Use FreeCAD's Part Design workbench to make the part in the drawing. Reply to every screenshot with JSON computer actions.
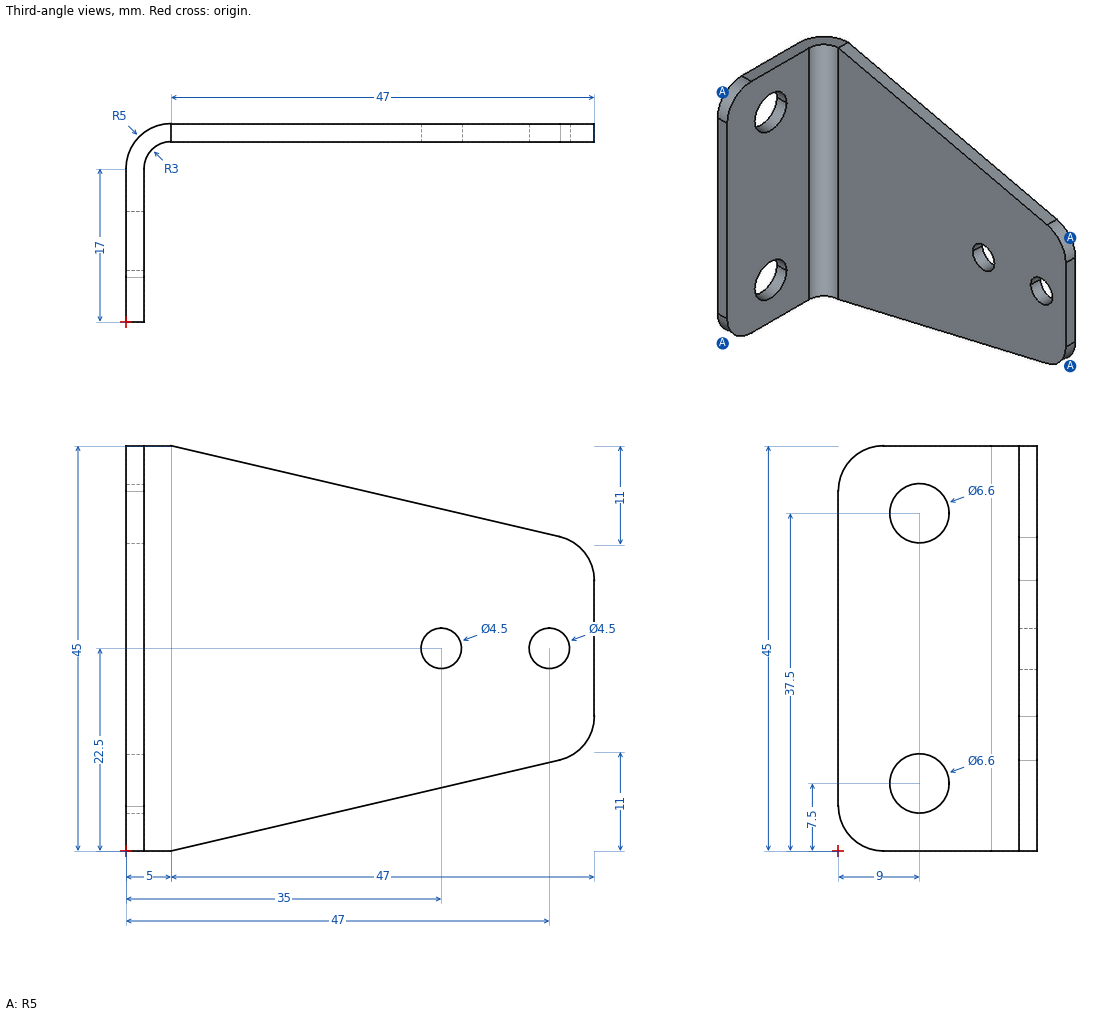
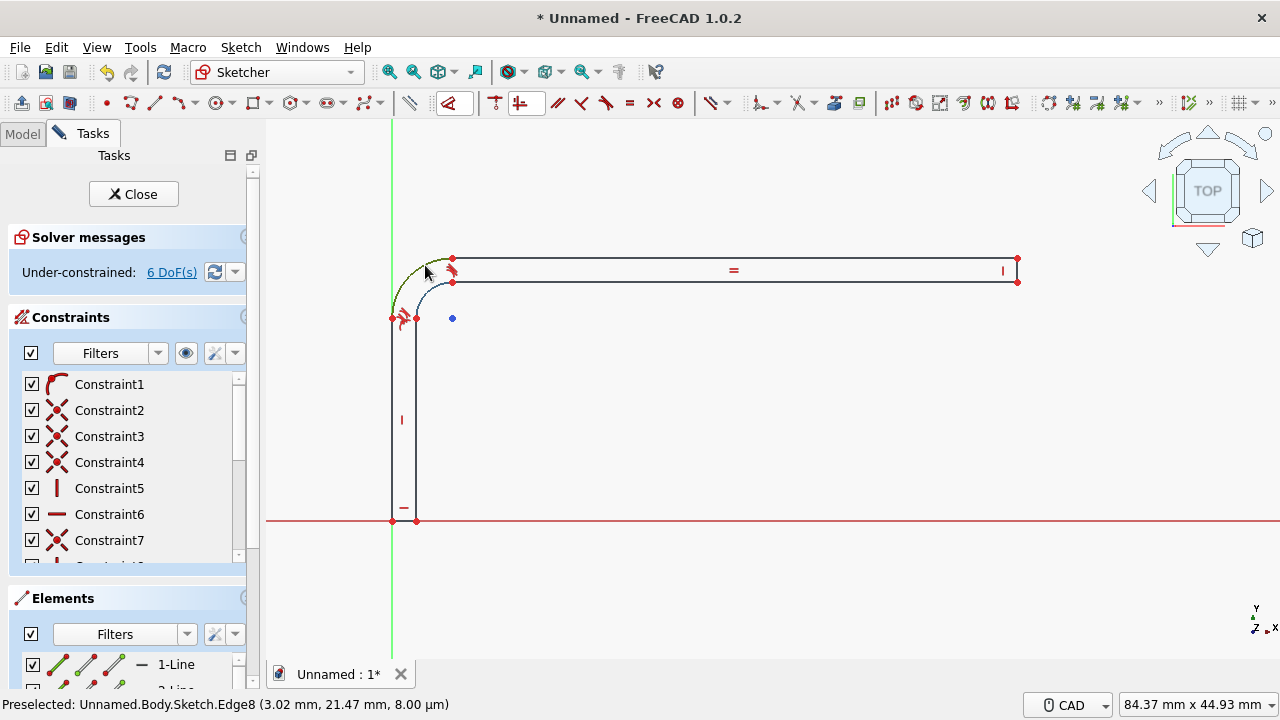
{"action": "key", "text": "c"}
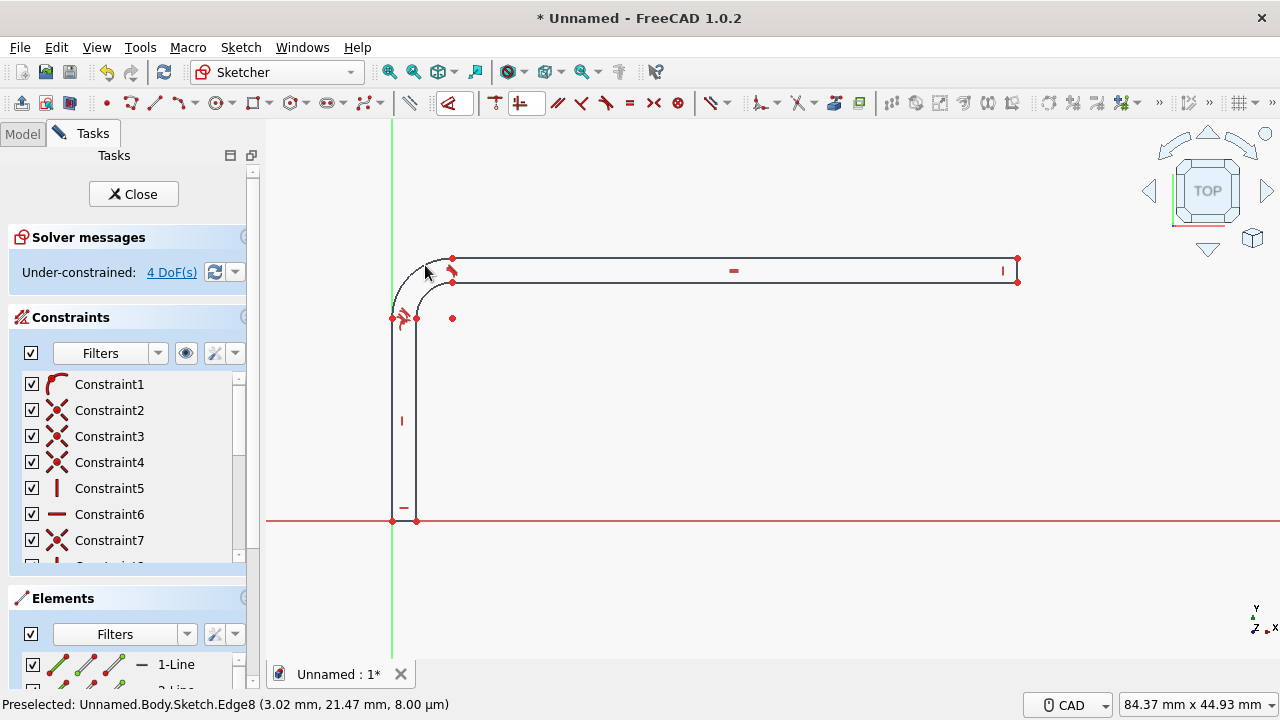
{"action": "left_click", "coordinate": [448, 104]}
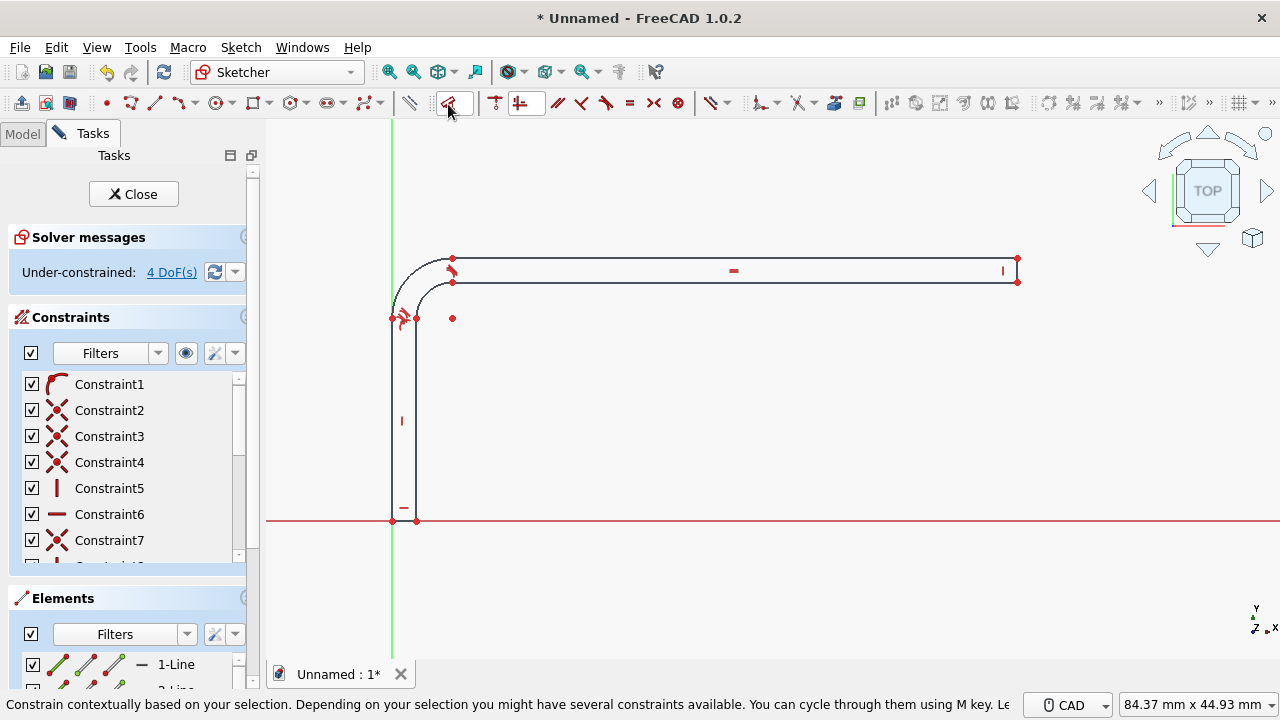
{"action": "left_click", "coordinate": [436, 287]}
{"action": "left_click", "coordinate": [484, 379]}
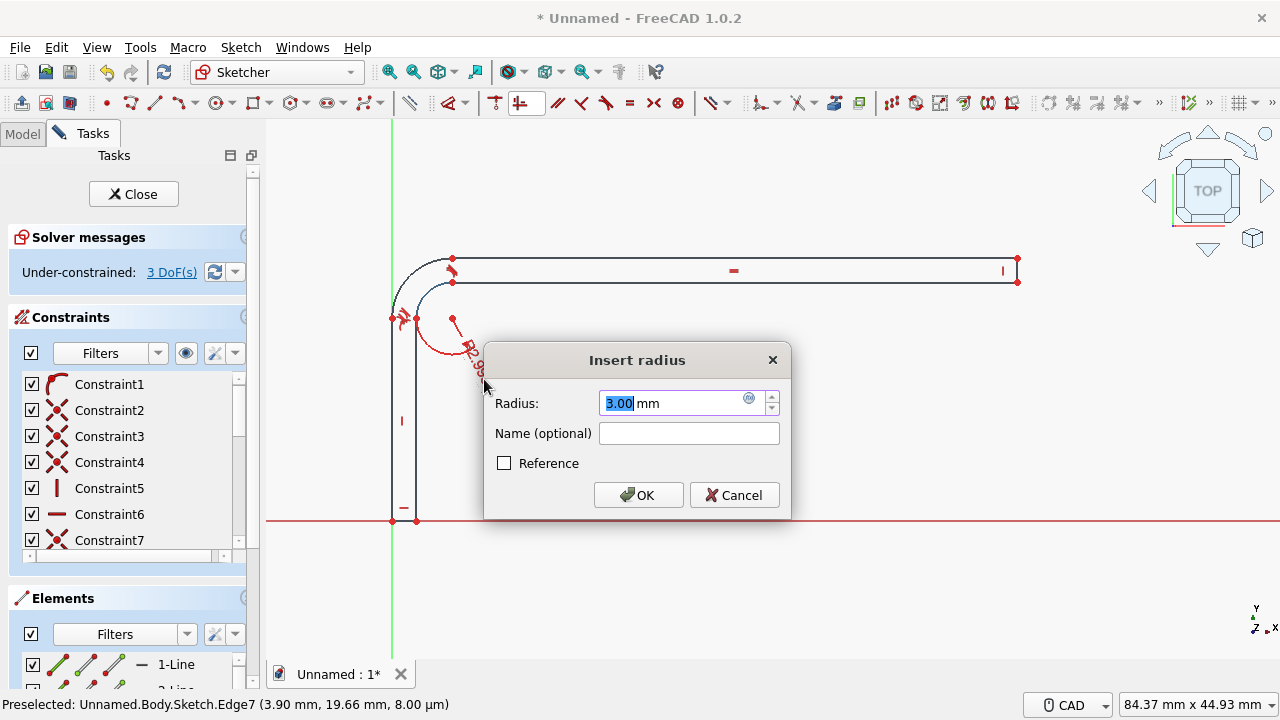
{"action": "type", "text": "3"}
{"action": "key", "text": "Return"}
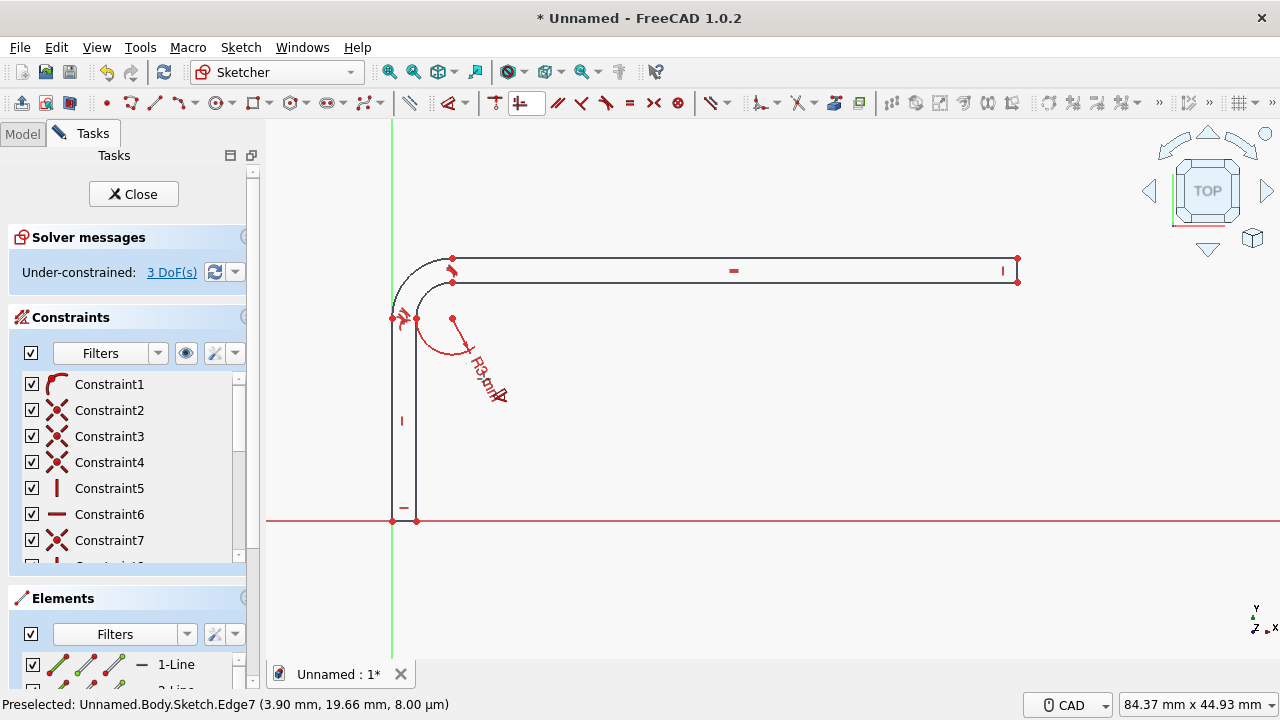
{"action": "left_click", "coordinate": [425, 265]}
{"action": "left_click", "coordinate": [410, 236]}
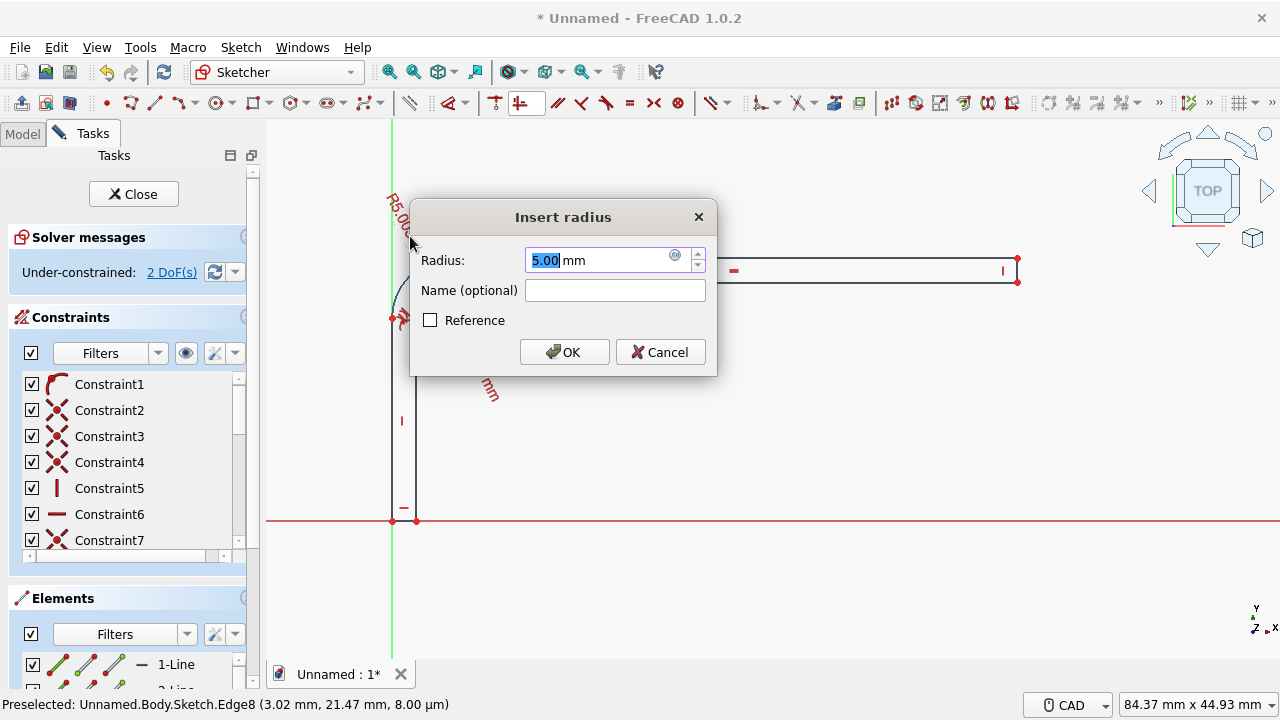
{"action": "type", "text": "5"}
{"action": "key", "text": "Return"}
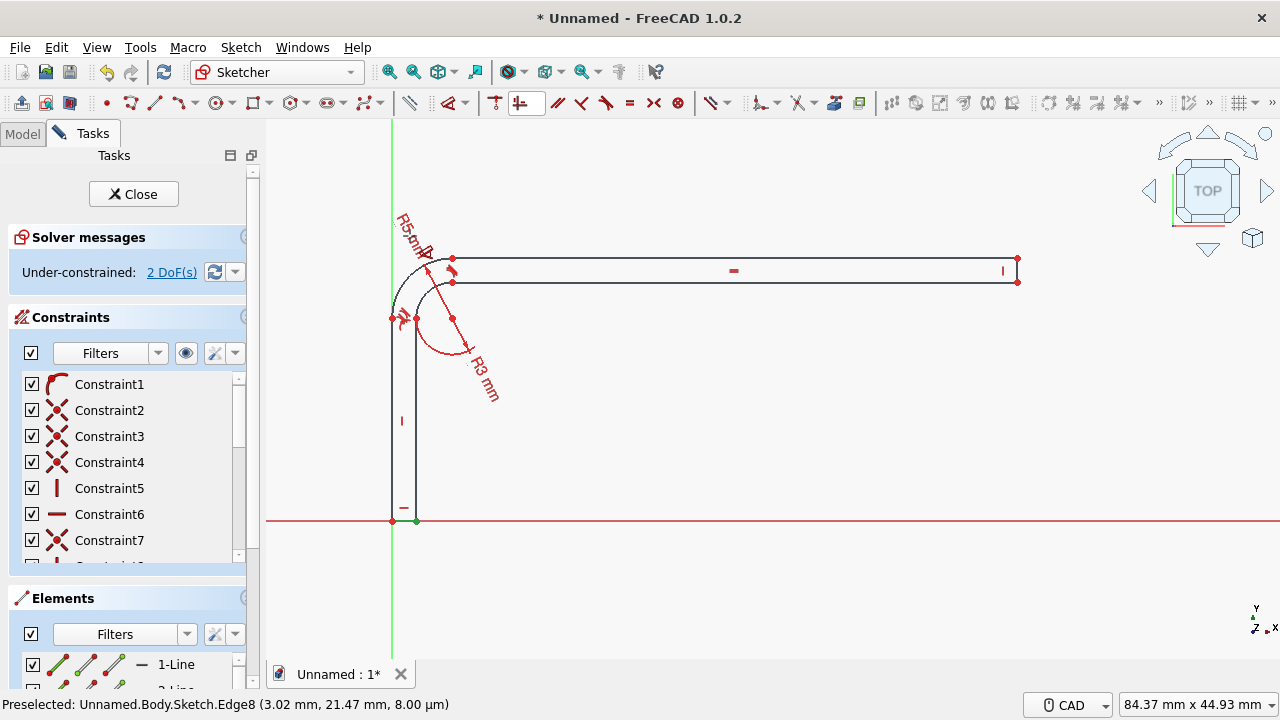
{"action": "left_click", "coordinate": [392, 379]}
{"action": "left_click", "coordinate": [358, 420]}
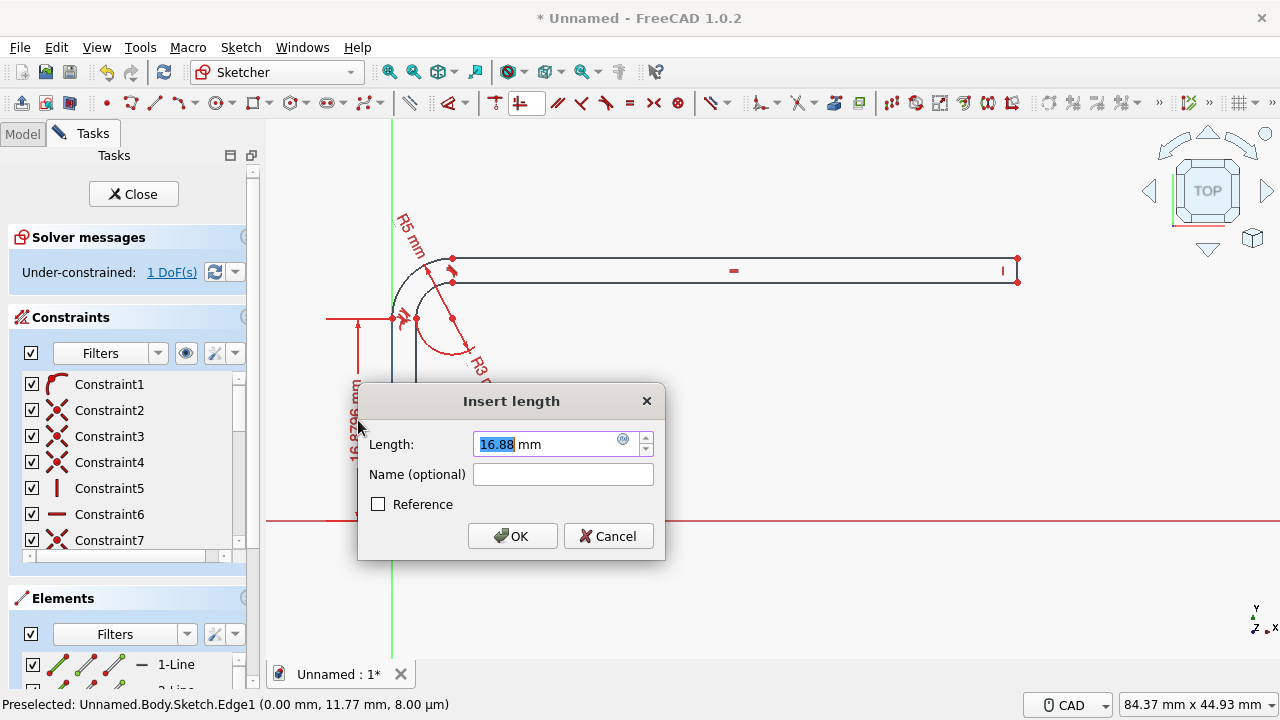
{"action": "type", "text": "17"}
{"action": "key", "text": "Return"}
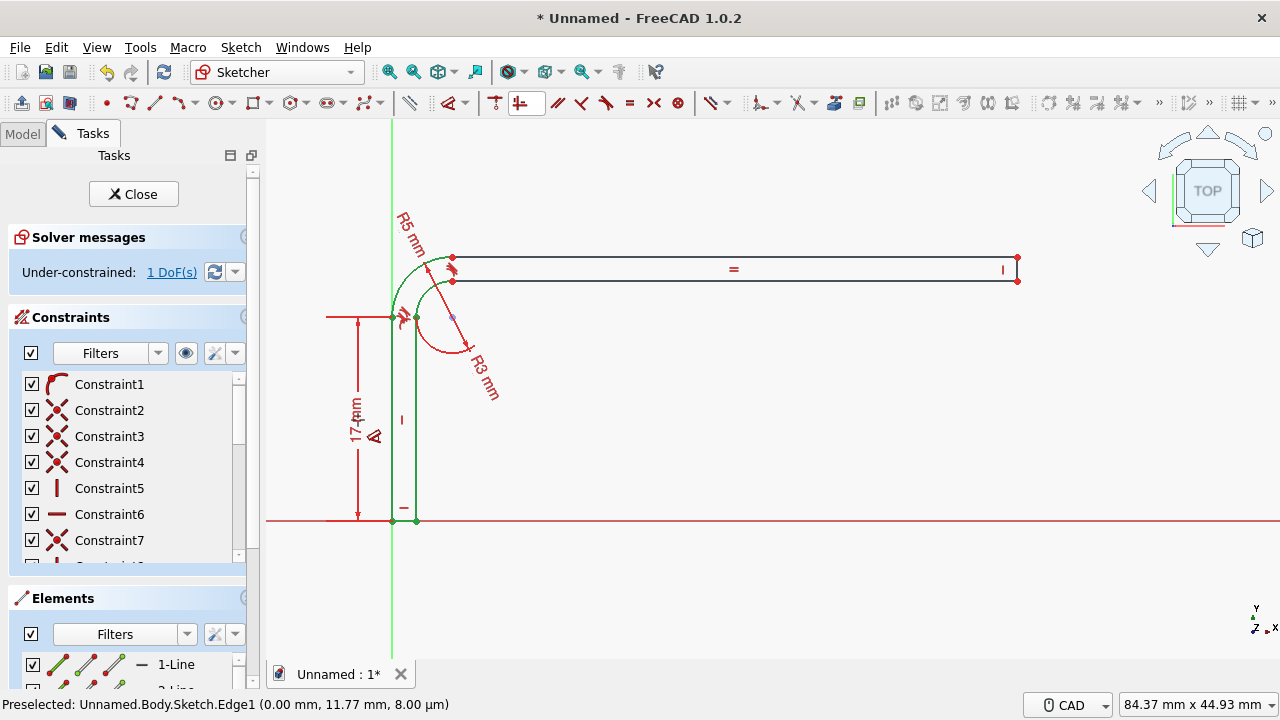
{"action": "left_click", "coordinate": [622, 281]}
{"action": "left_click", "coordinate": [735, 315]}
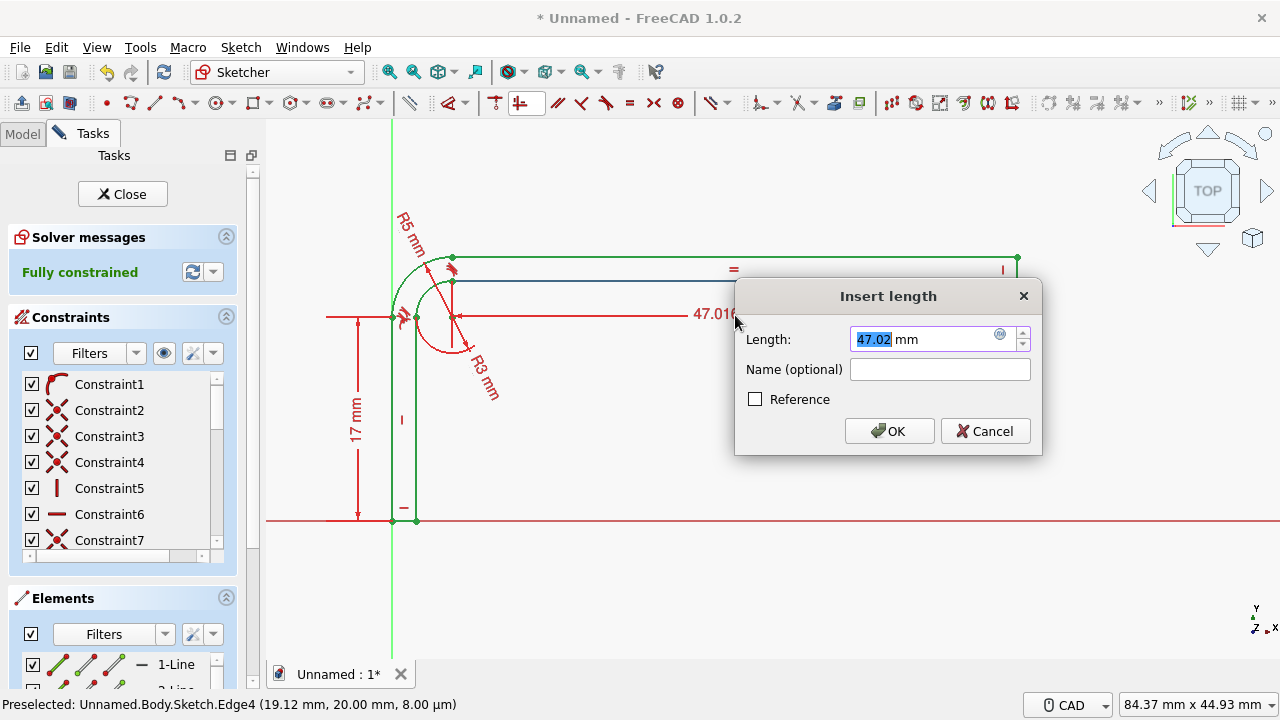
{"action": "type", "text": "47"}
{"action": "key", "text": "Return"}
{"action": "key", "text": "Escape"}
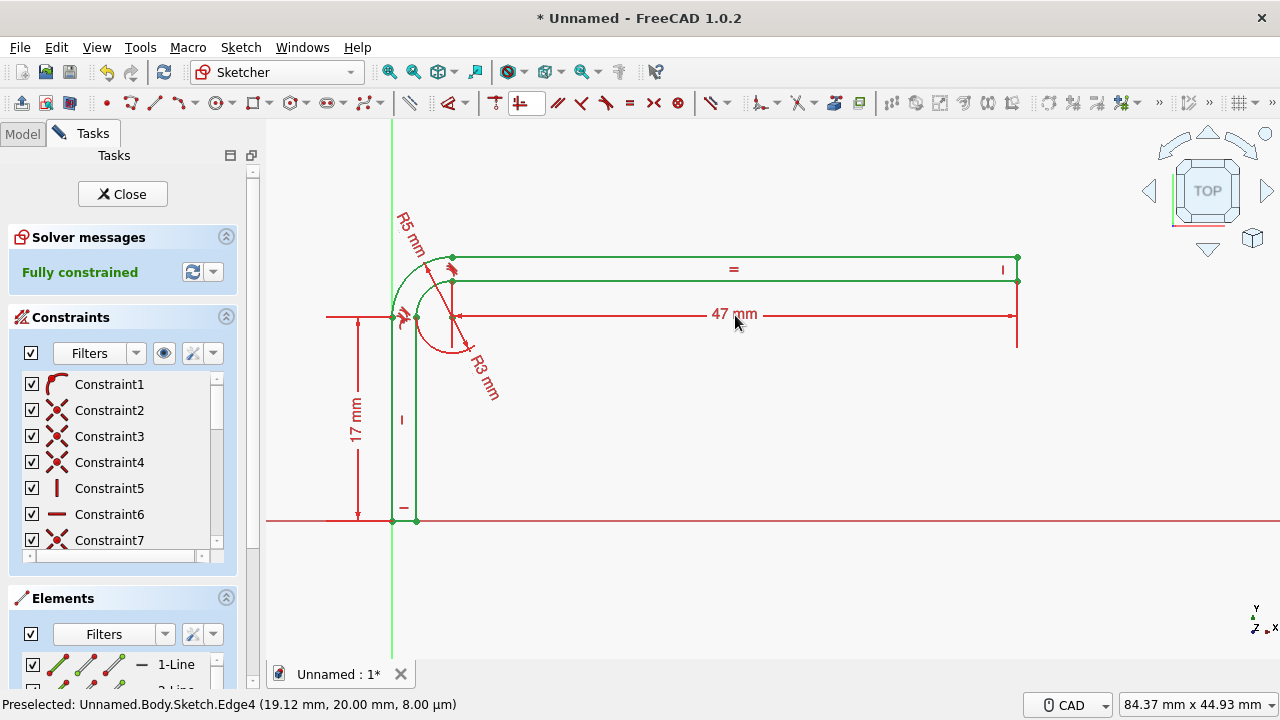
{"action": "left_click", "coordinate": [123, 194]}